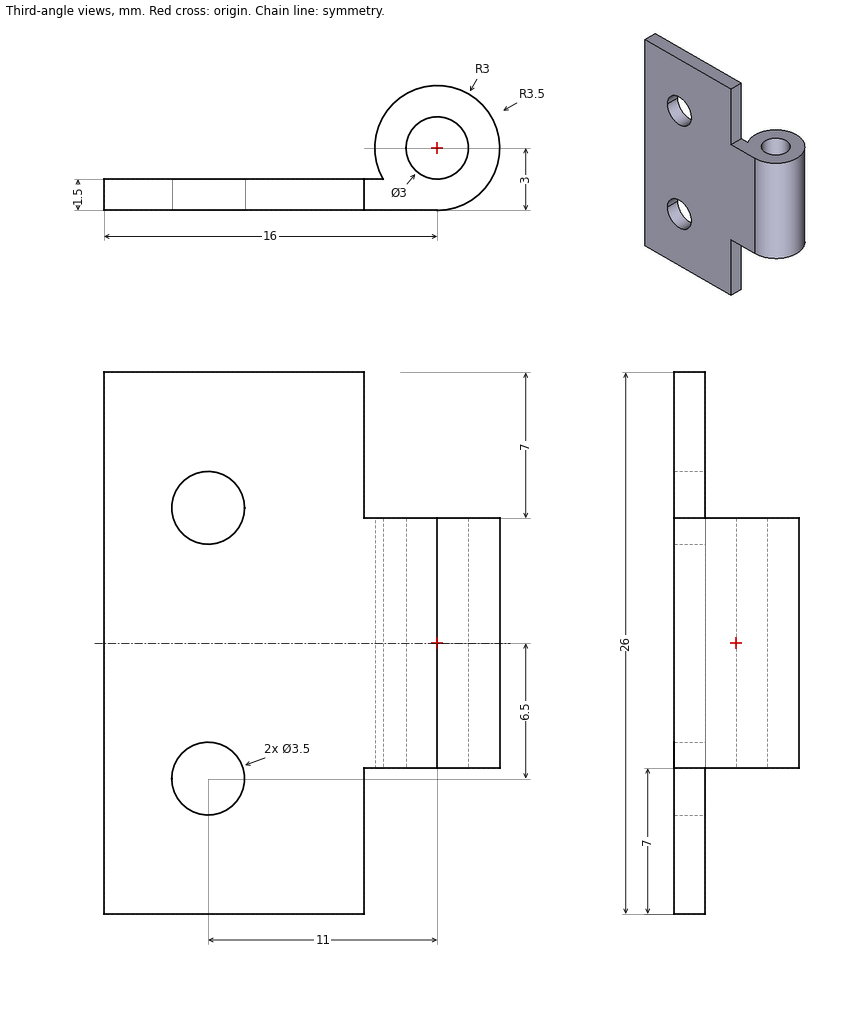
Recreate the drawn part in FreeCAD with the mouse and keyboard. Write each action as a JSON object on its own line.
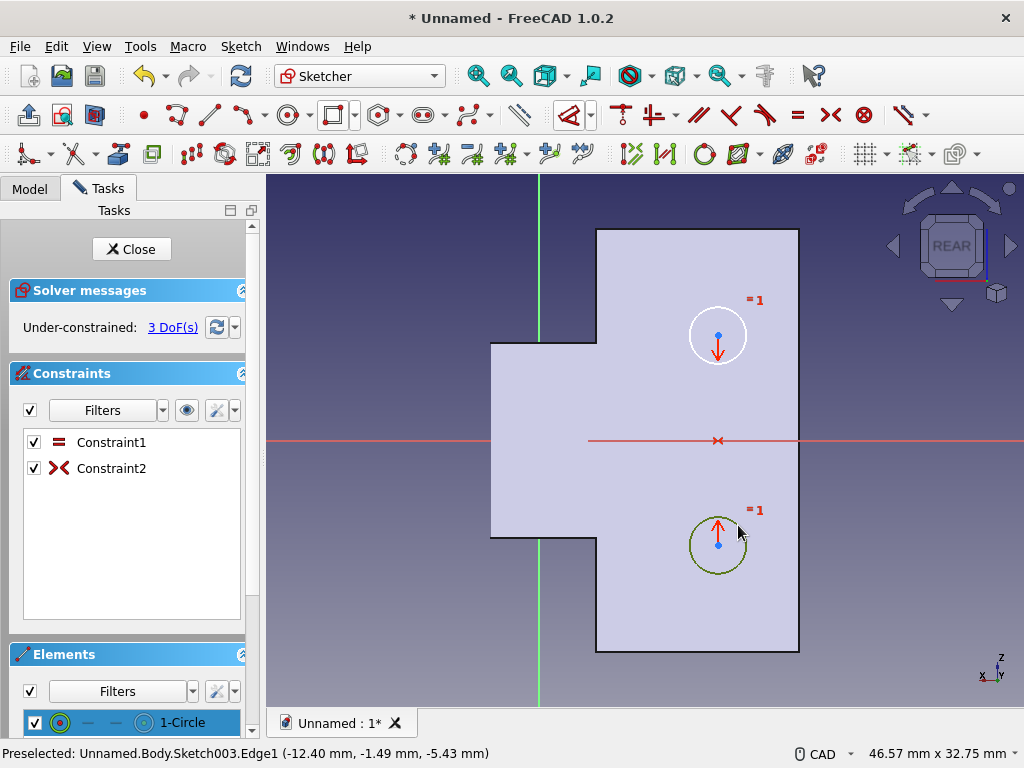
{"action": "key", "text": "k o"}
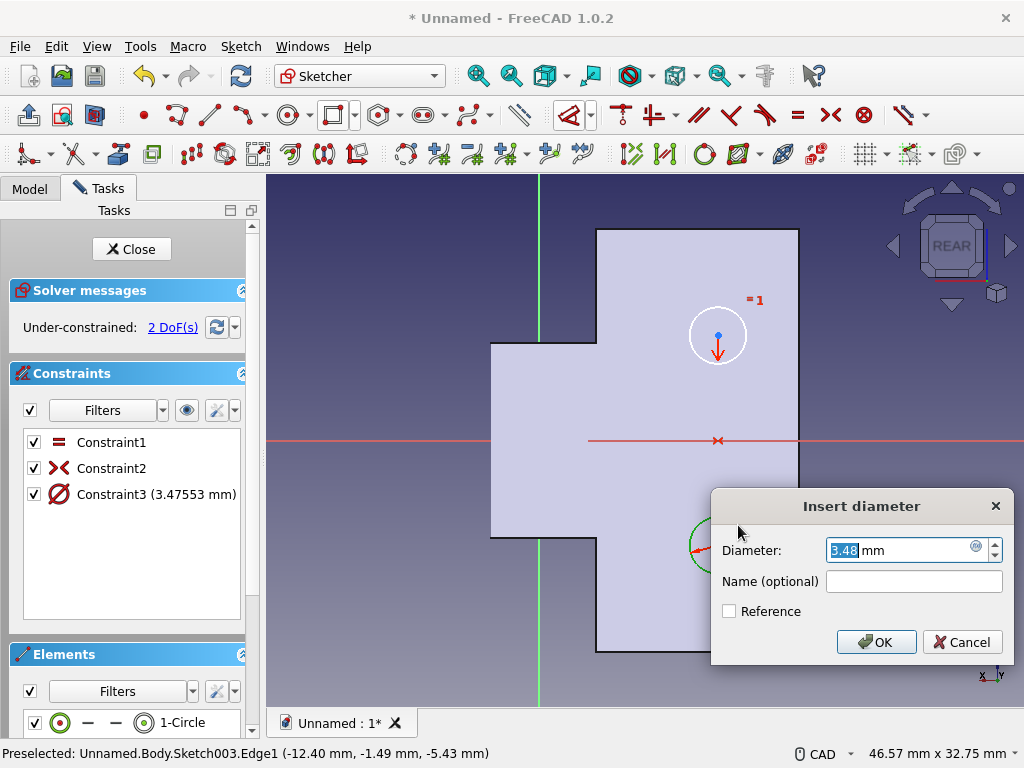
{"action": "type", "text": "3.5"}
{"action": "key", "text": "Return"}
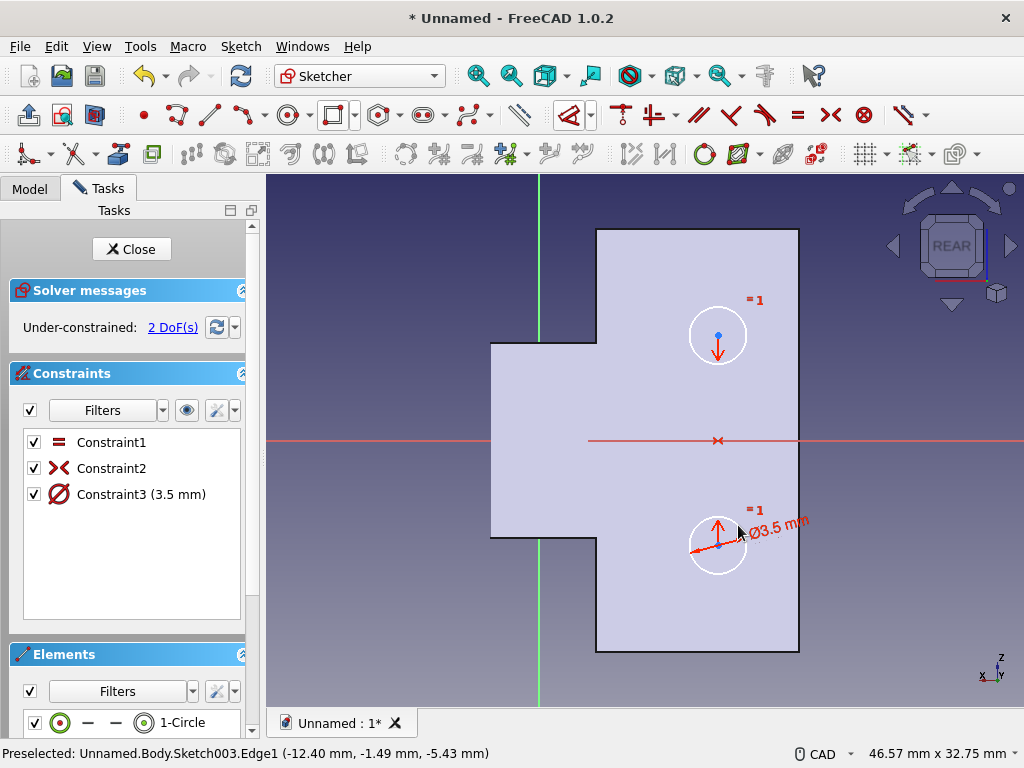
{"action": "left_click", "coordinate": [718, 545]}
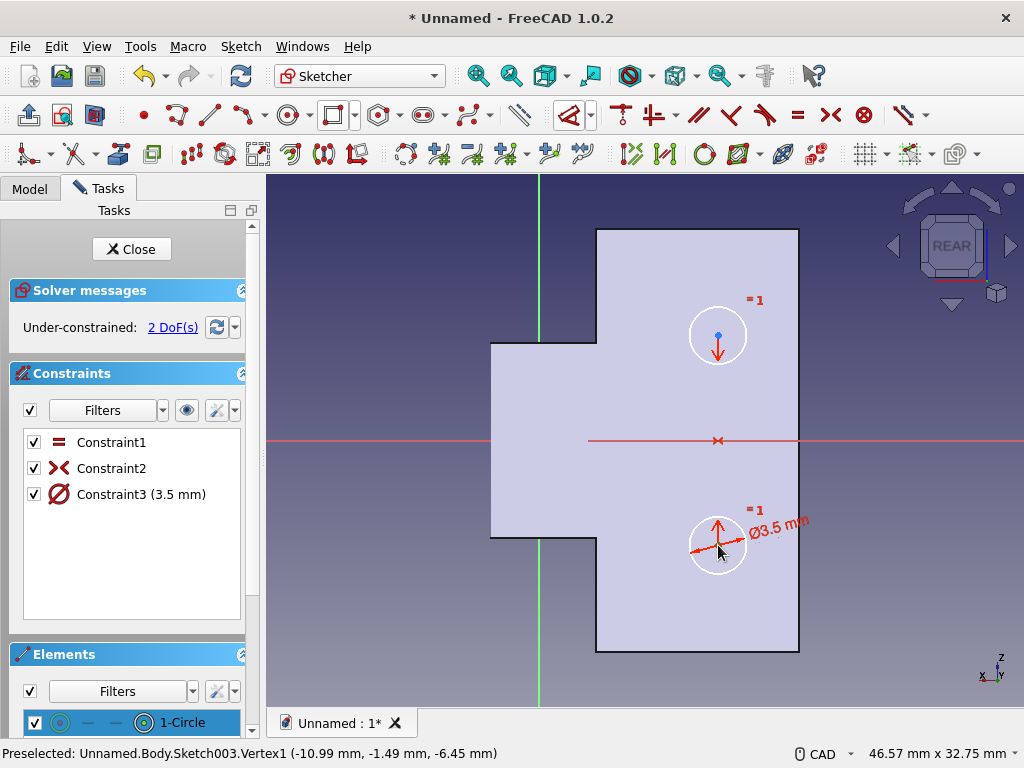
{"action": "left_click", "coordinate": [590, 116]}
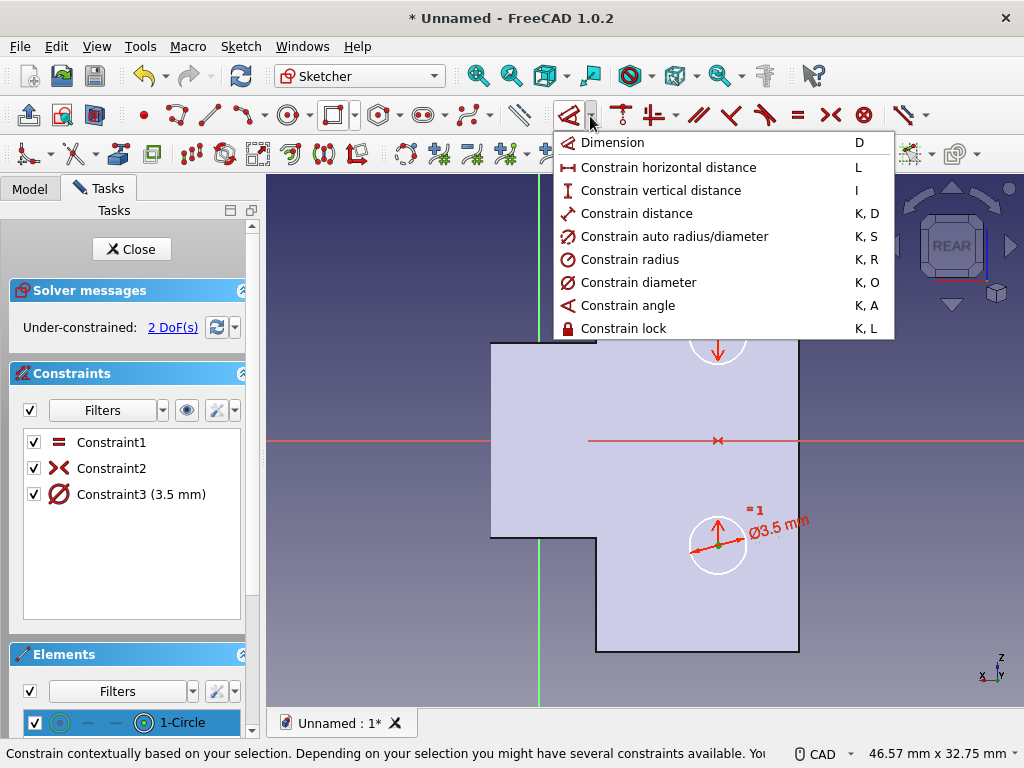
{"action": "left_click", "coordinate": [724, 168]}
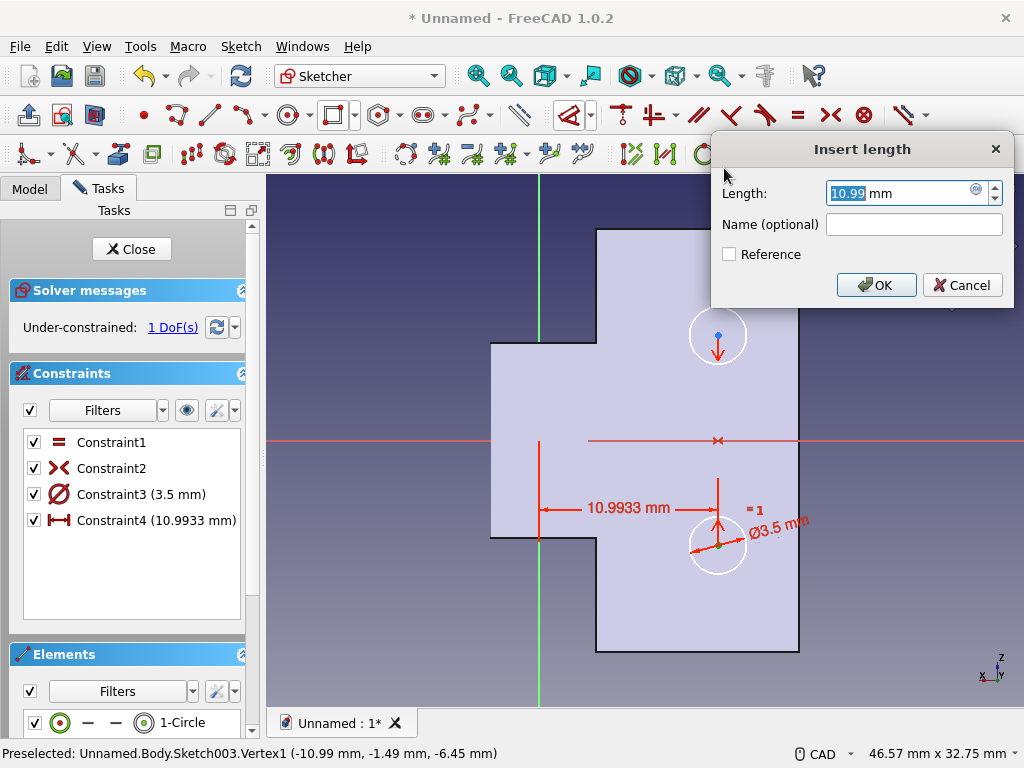
{"action": "type", "text": "11"}
{"action": "key", "text": "Return"}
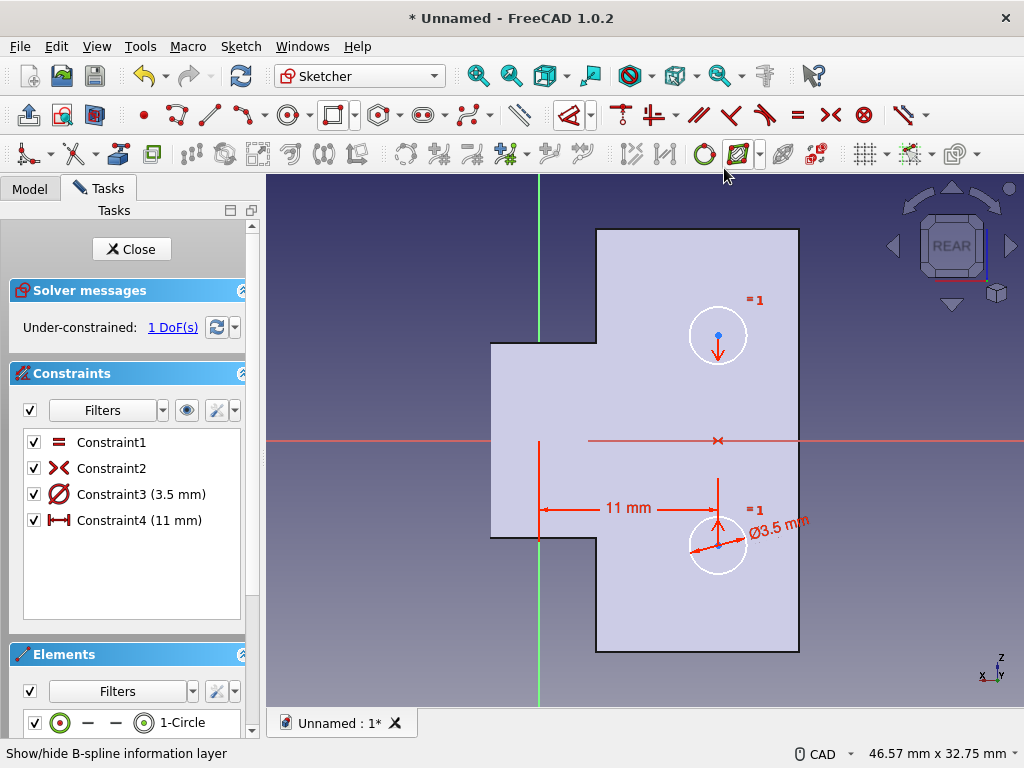
{"action": "left_click", "coordinate": [718, 545]}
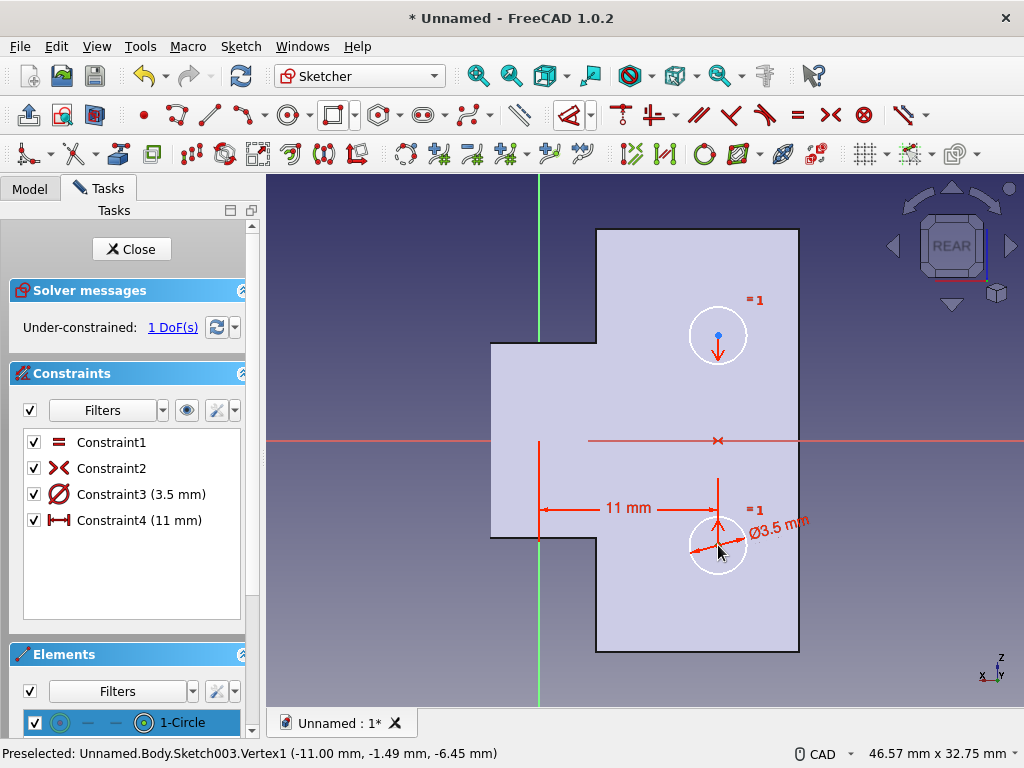
{"action": "left_click", "coordinate": [590, 116]}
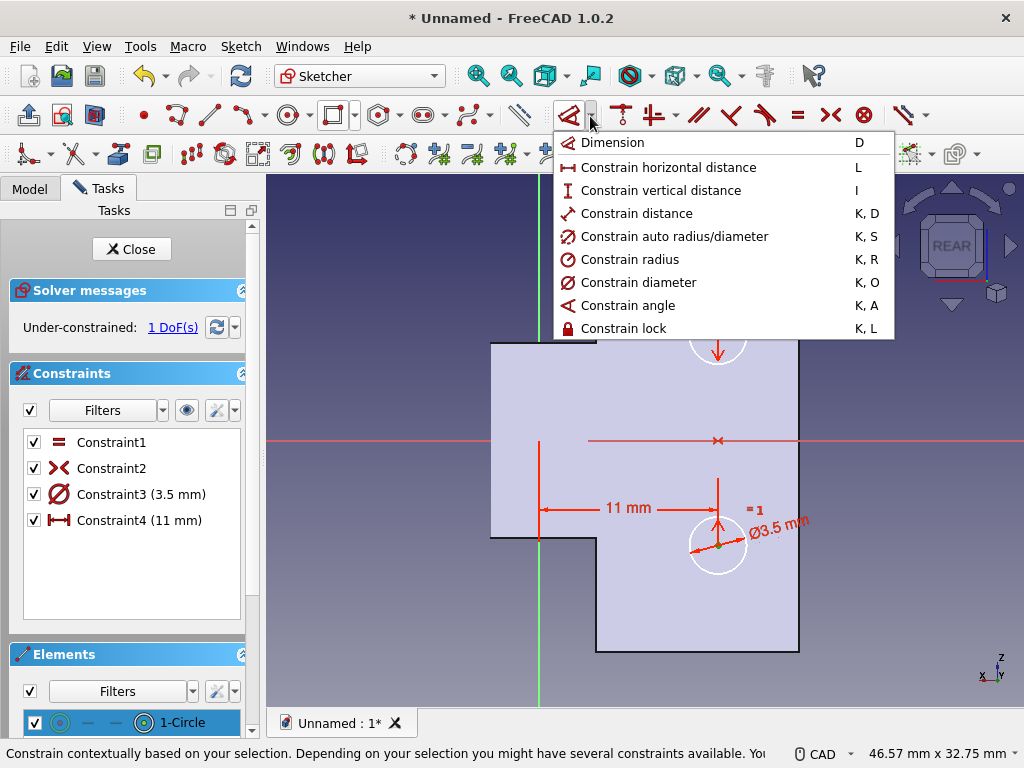
{"action": "left_click", "coordinate": [724, 190]}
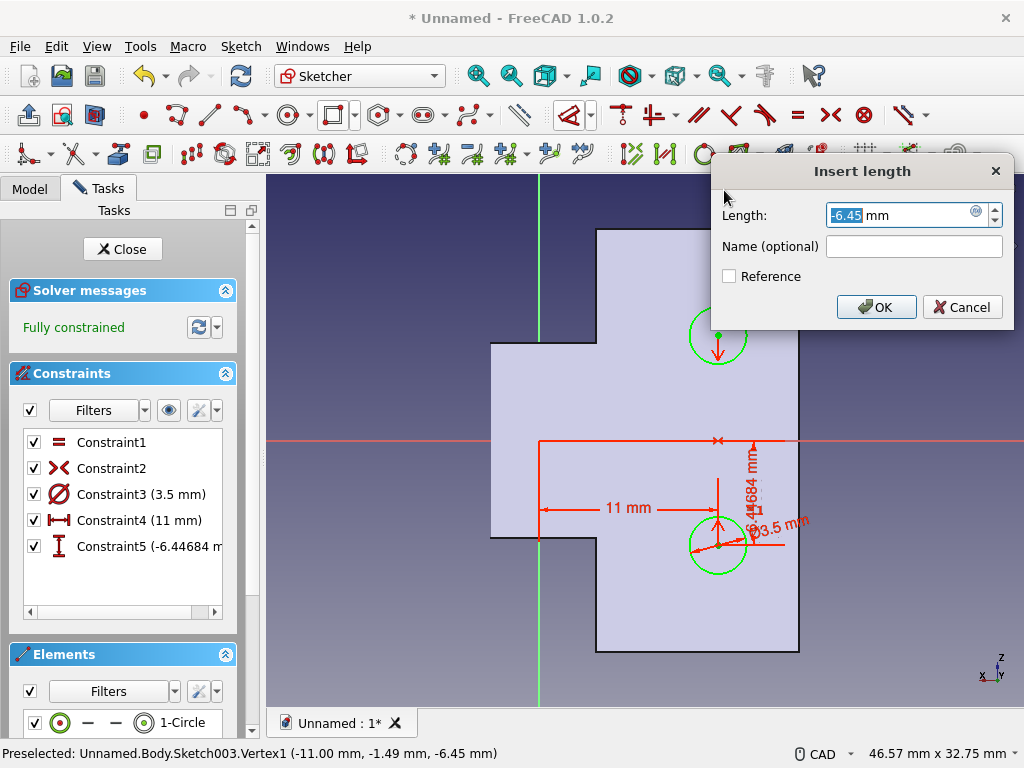
{"action": "type", "text": "-6.5"}
{"action": "key", "text": "Return"}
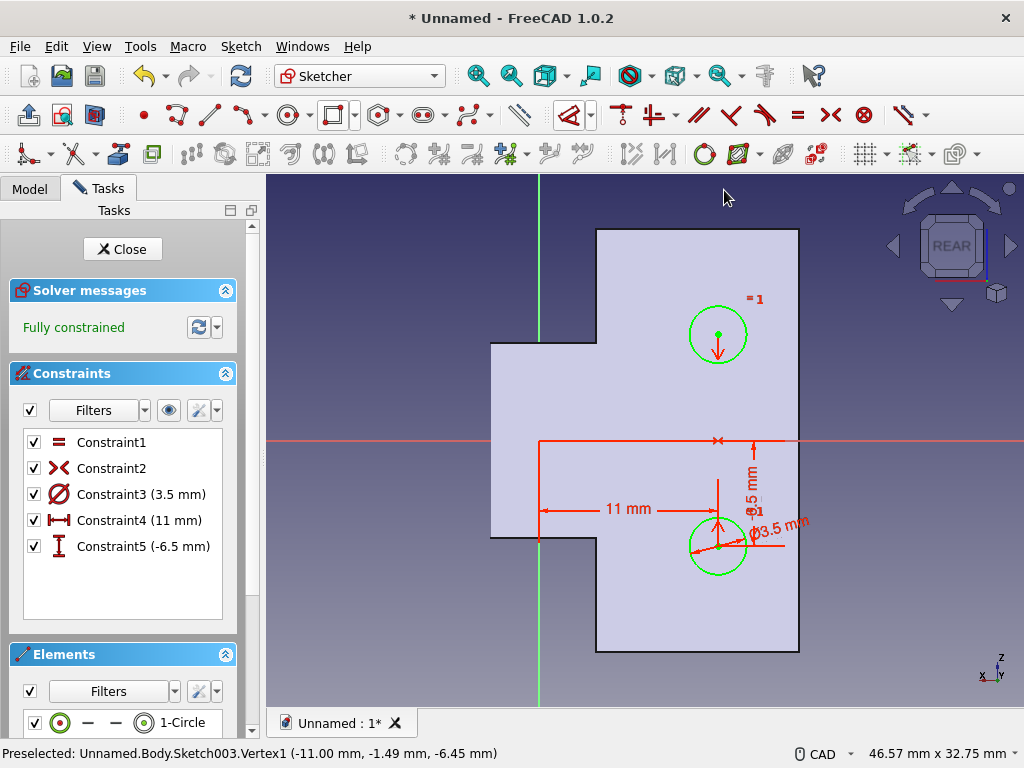
{"action": "left_click", "coordinate": [123, 249]}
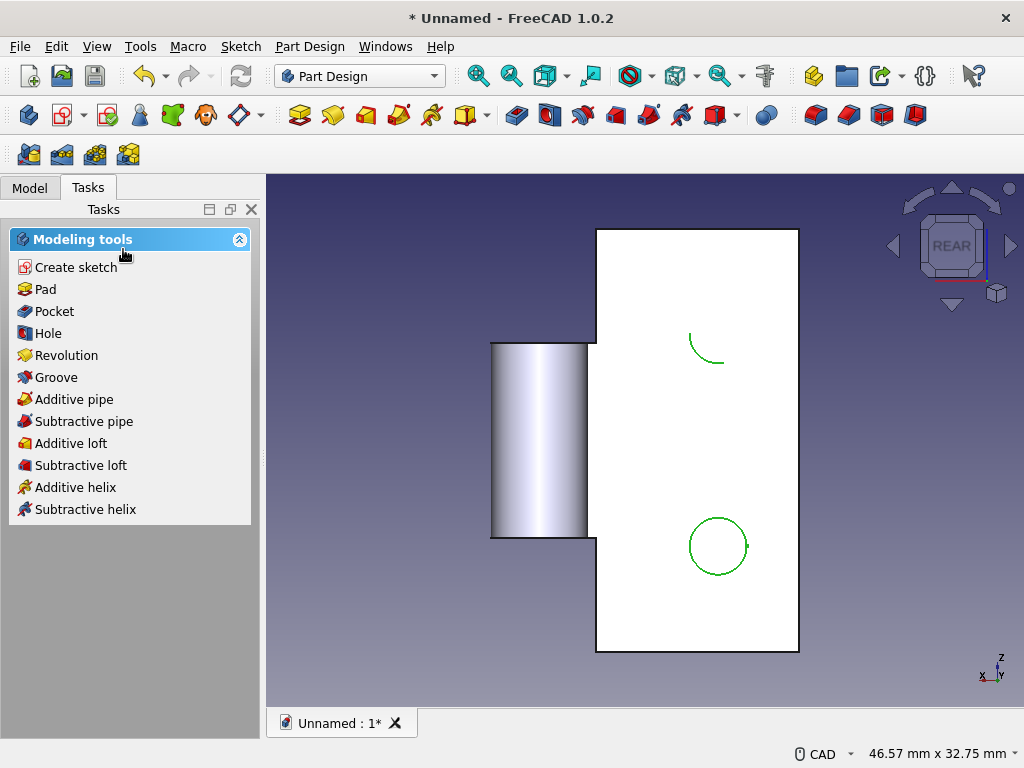
{"action": "left_click", "coordinate": [517, 116]}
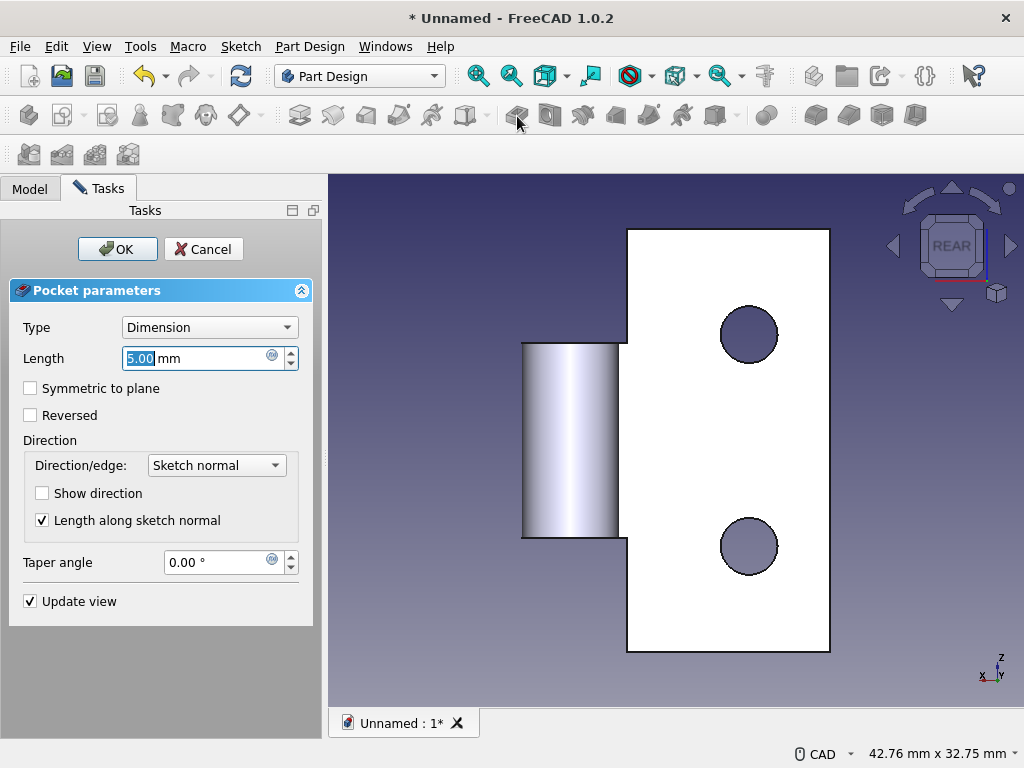
{"action": "left_click", "coordinate": [210, 328]}